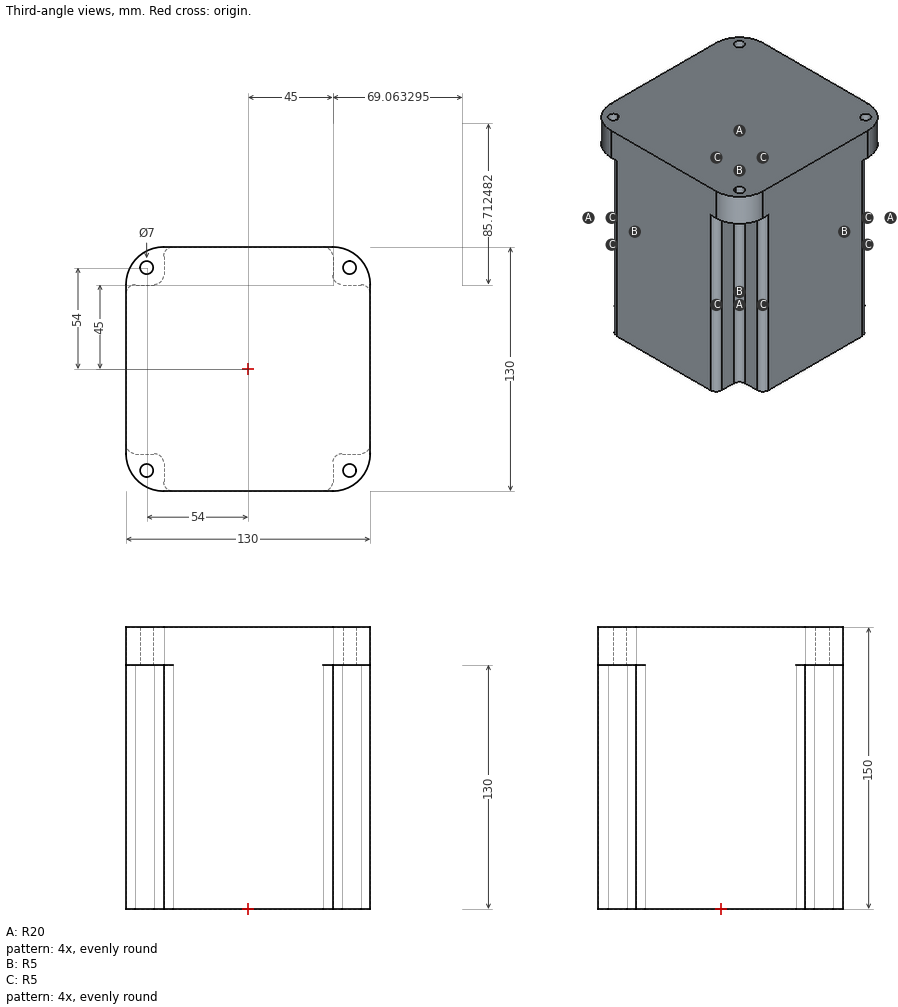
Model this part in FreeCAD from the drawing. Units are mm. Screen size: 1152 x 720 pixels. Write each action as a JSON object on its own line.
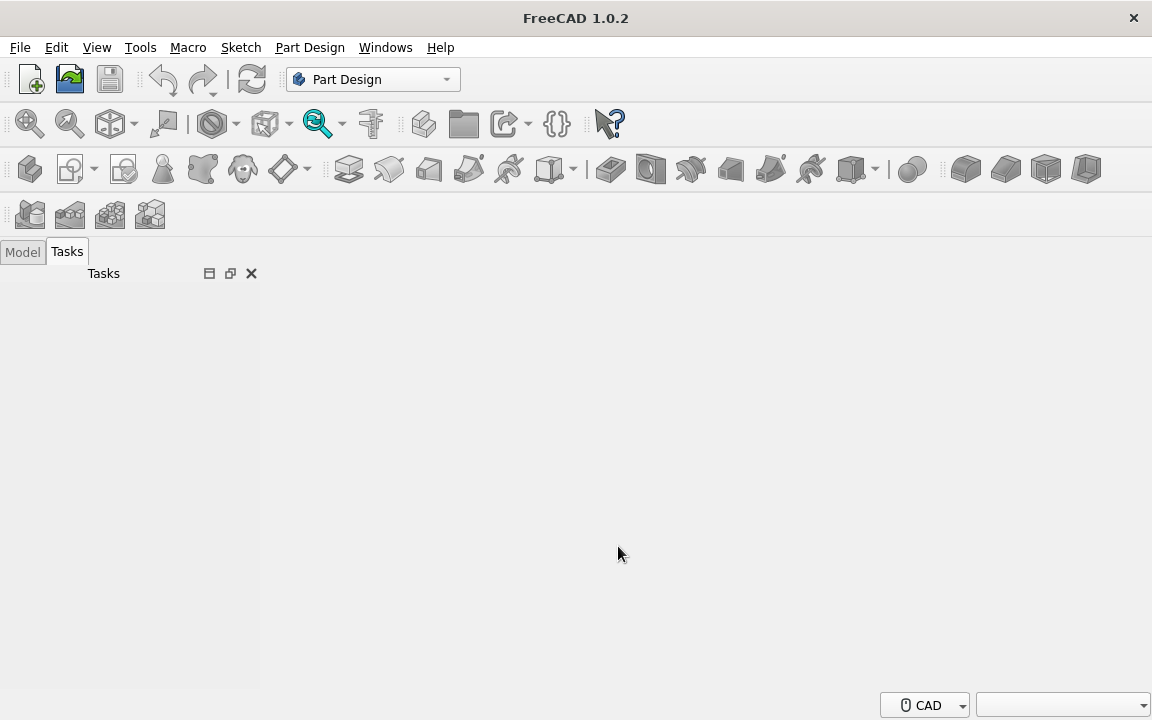
{"action": "key", "text": "ctrl+n"}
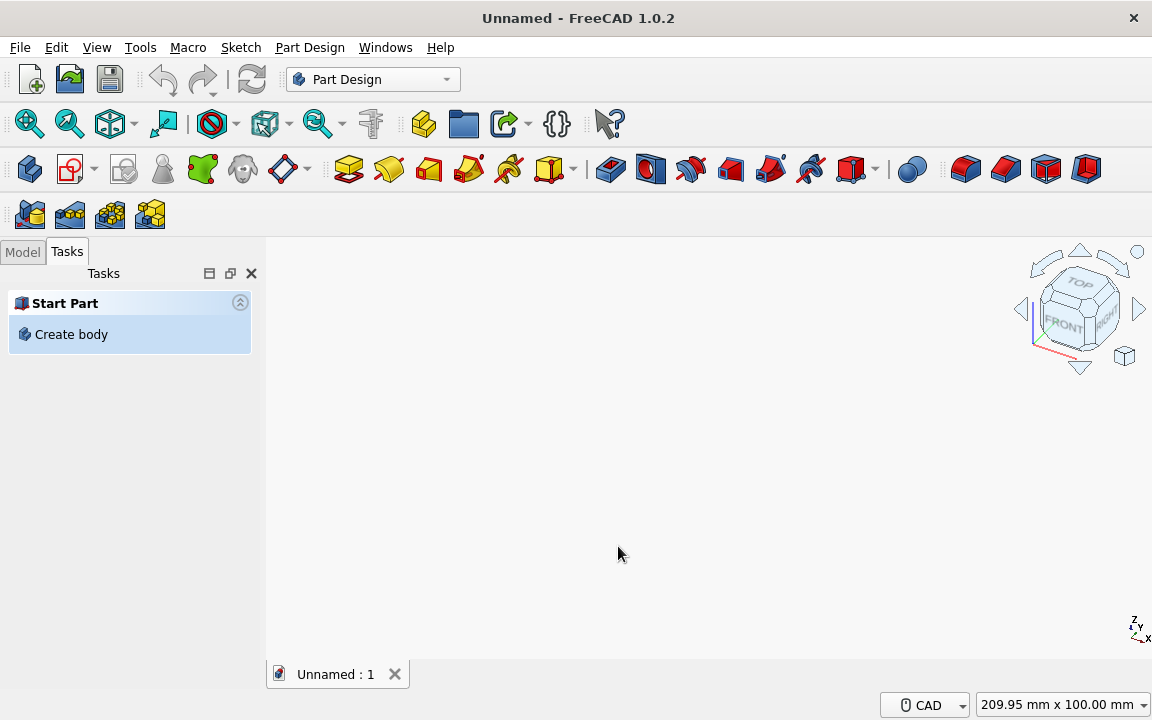
{"action": "left_click", "coordinate": [70, 170]}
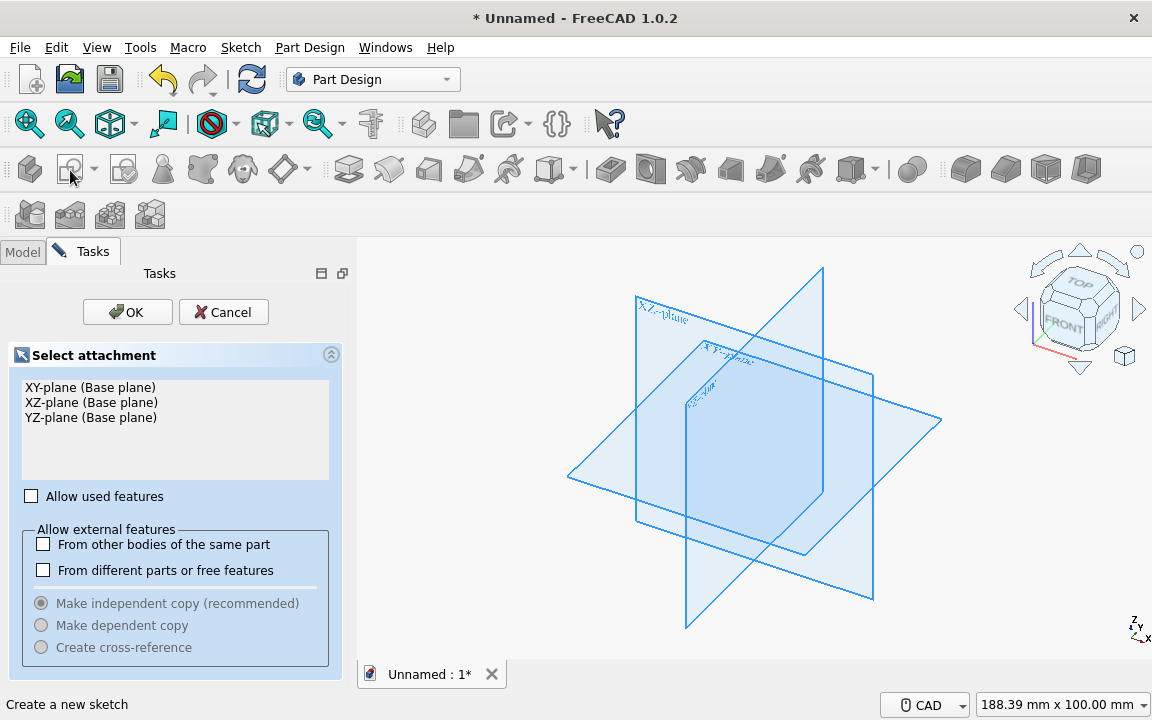
{"action": "left_click", "coordinate": [82, 388]}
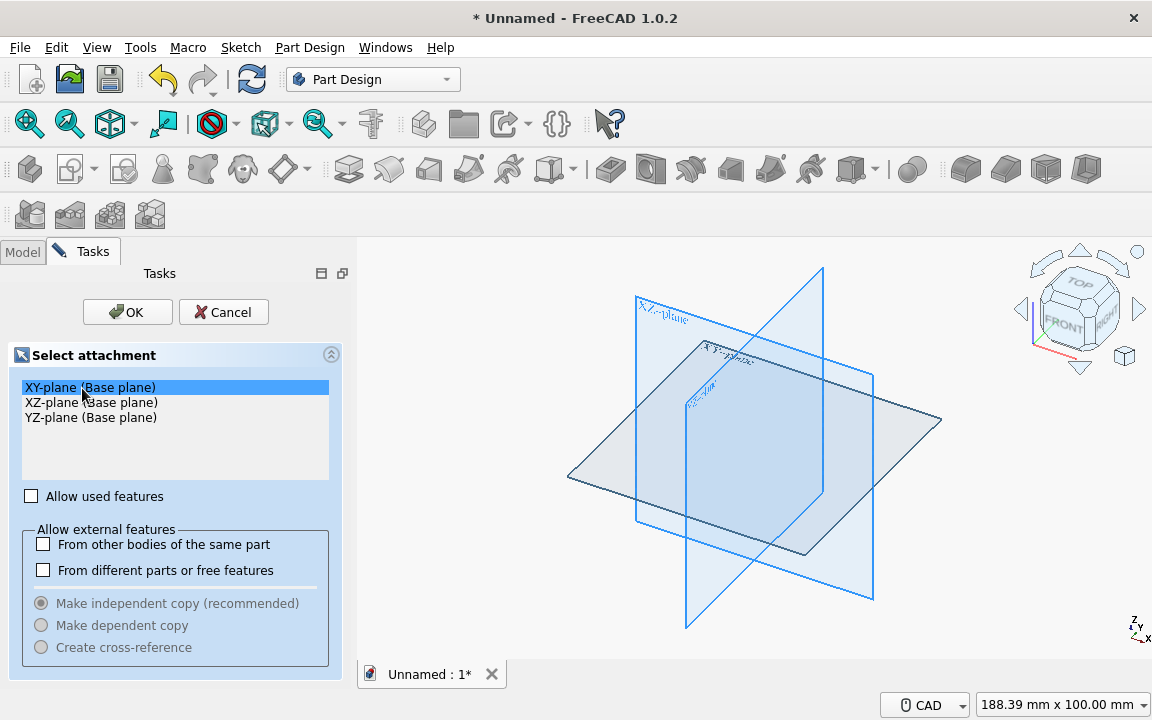
{"action": "left_click", "coordinate": [128, 312]}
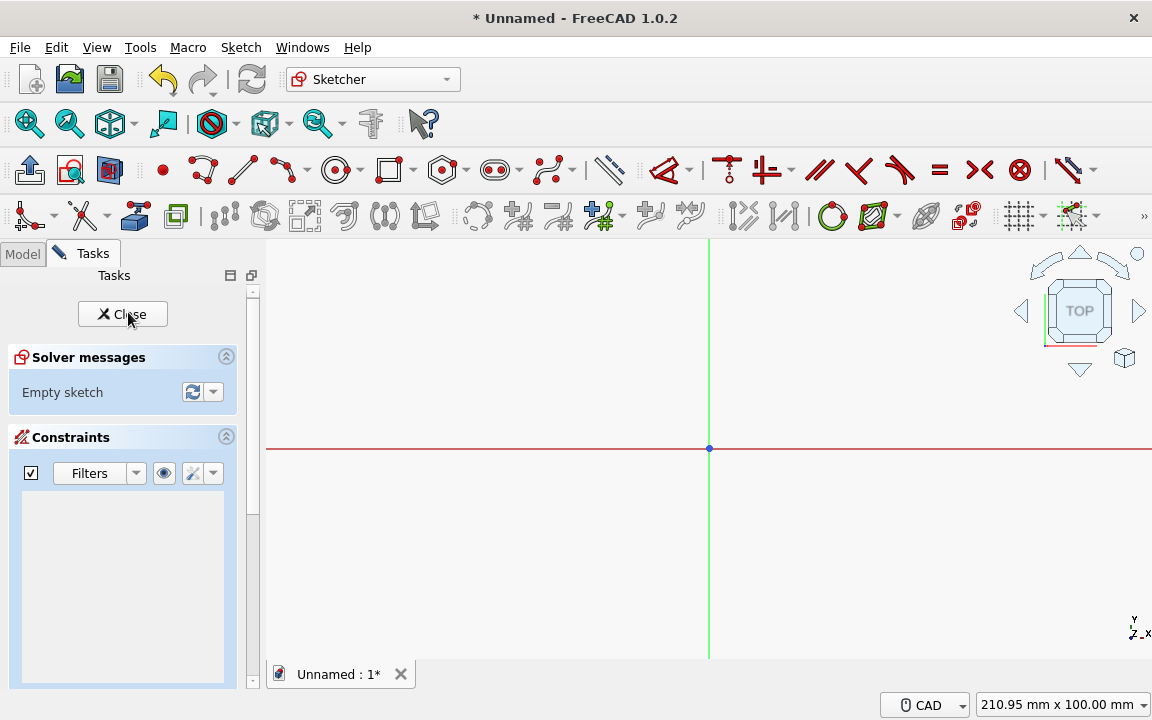
{"action": "scroll", "coordinate": [585, 449], "scroll_direction": "down", "scroll_amount": 4}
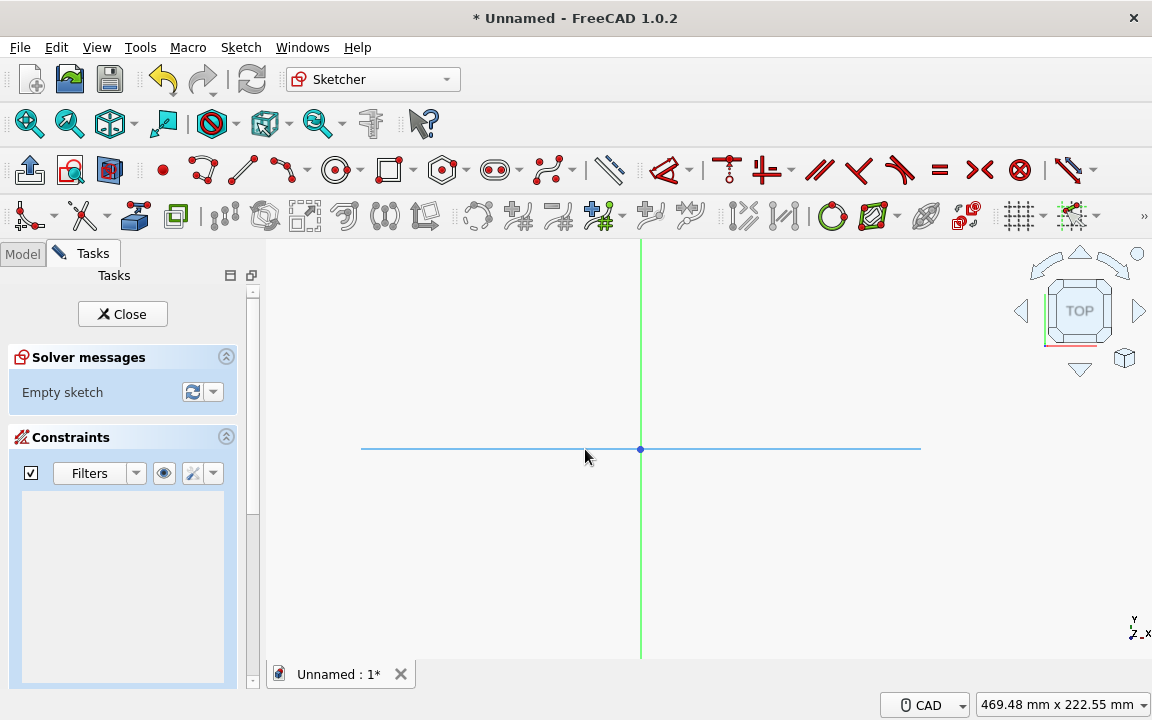
{"action": "key", "text": "g v"}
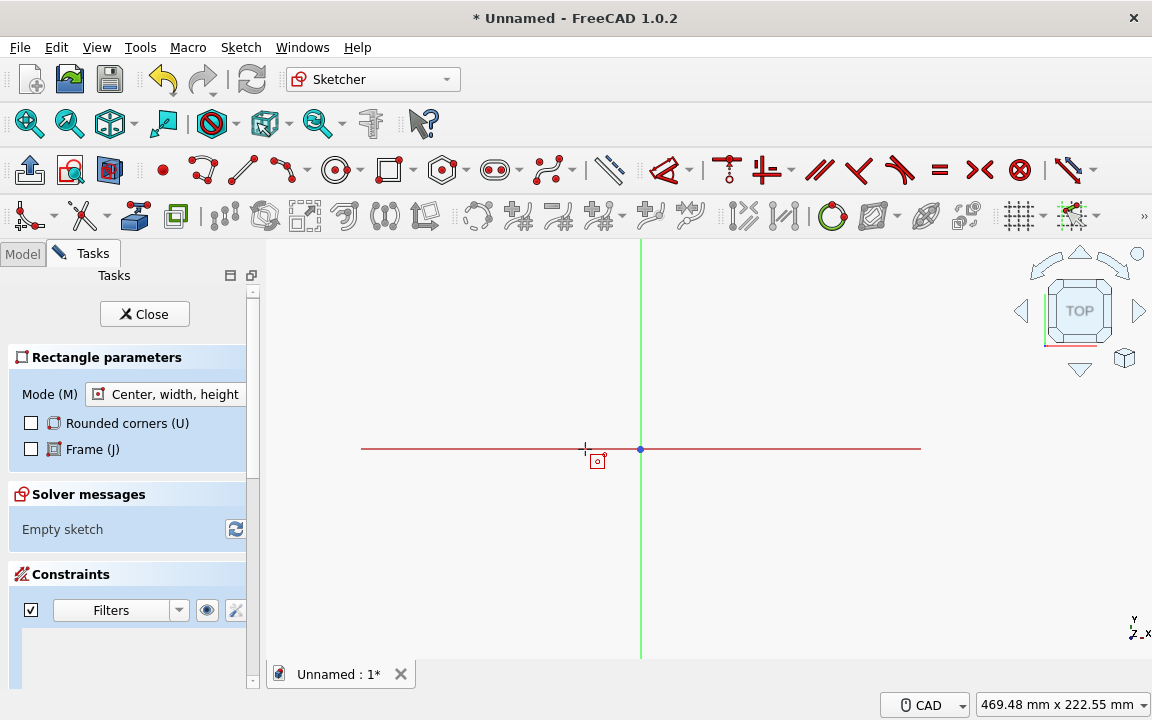
{"action": "left_click", "coordinate": [641, 449]}
{"action": "mouse_move", "coordinate": [764, 327]}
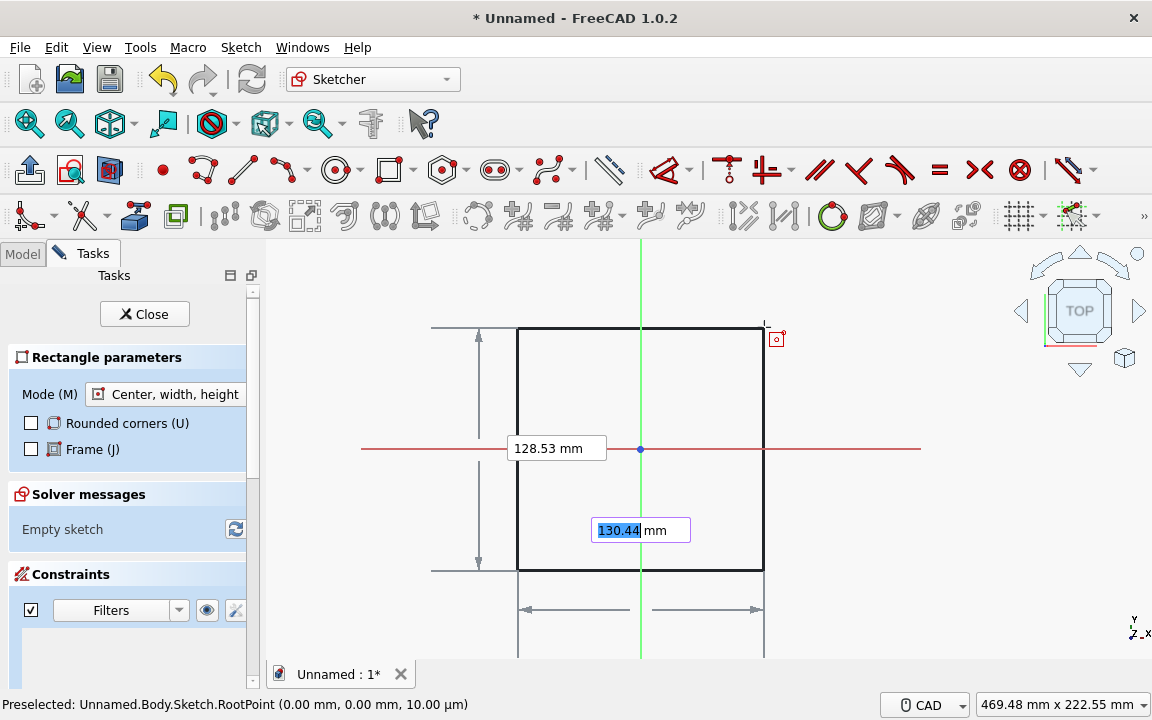
{"action": "type", "text": "130"}
{"action": "key", "text": "Tab"}
{"action": "type", "text": "130"}
{"action": "key", "text": "Return"}
{"action": "key", "text": "Escape"}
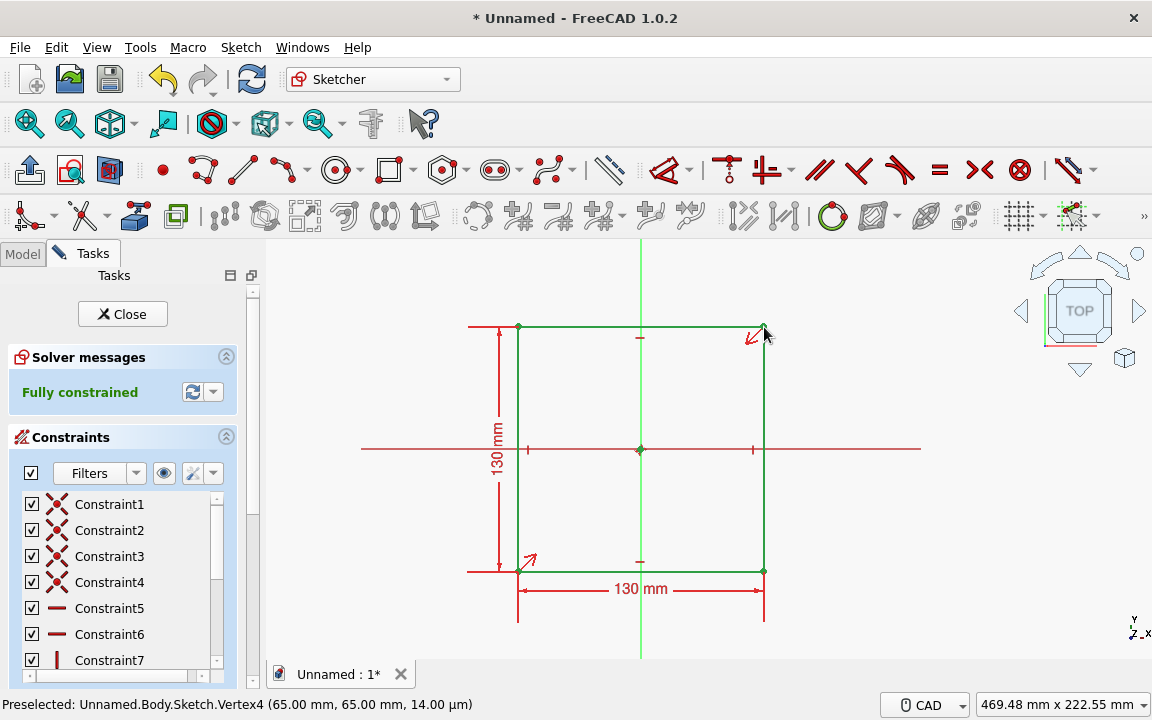
{"action": "left_click", "coordinate": [123, 314]}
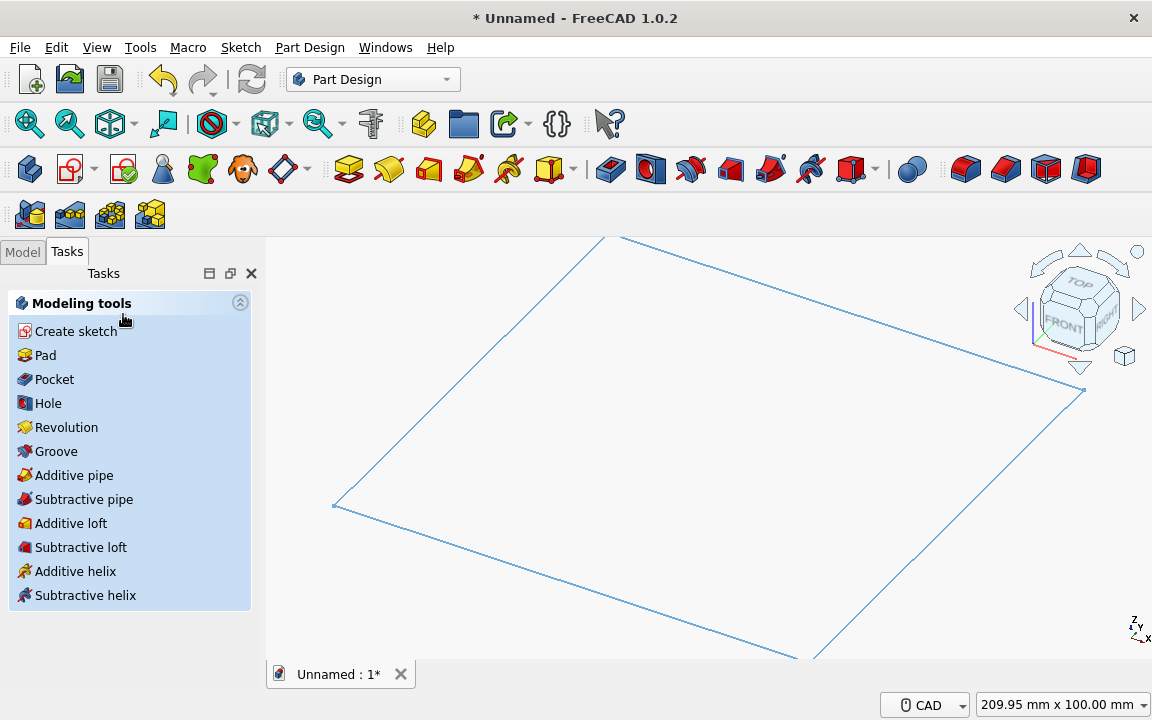
{"action": "left_click", "coordinate": [350, 170]}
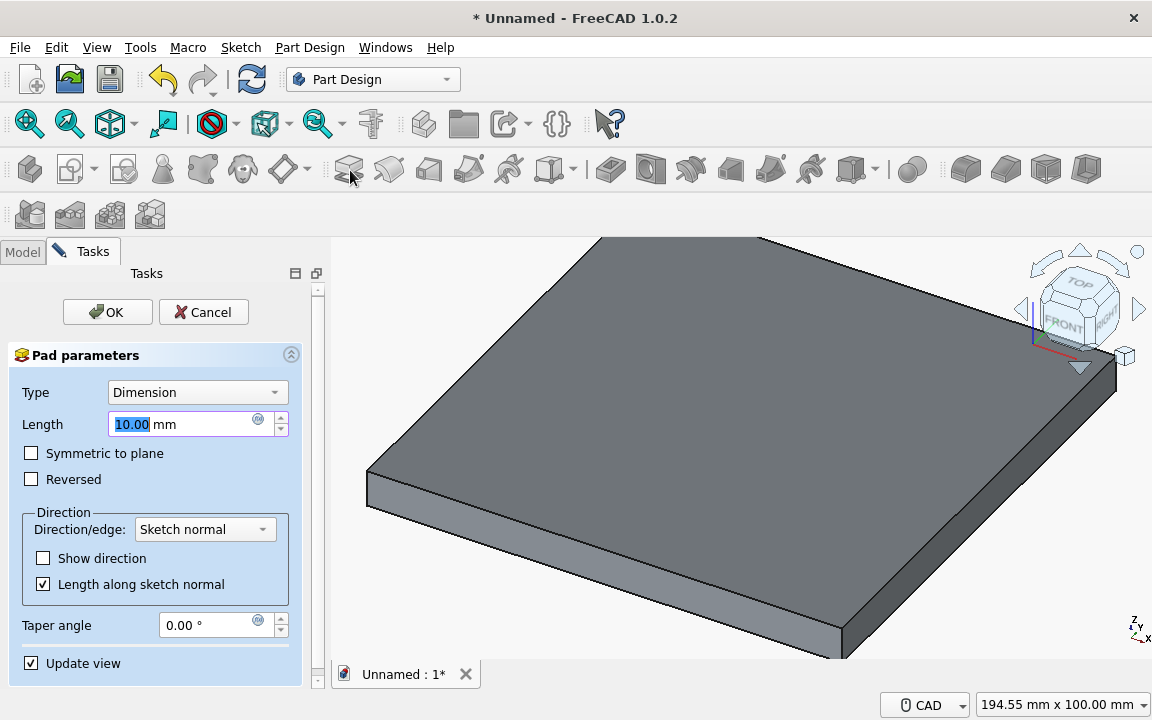
{"action": "type", "text": "150"}
{"action": "key", "text": "Tab"}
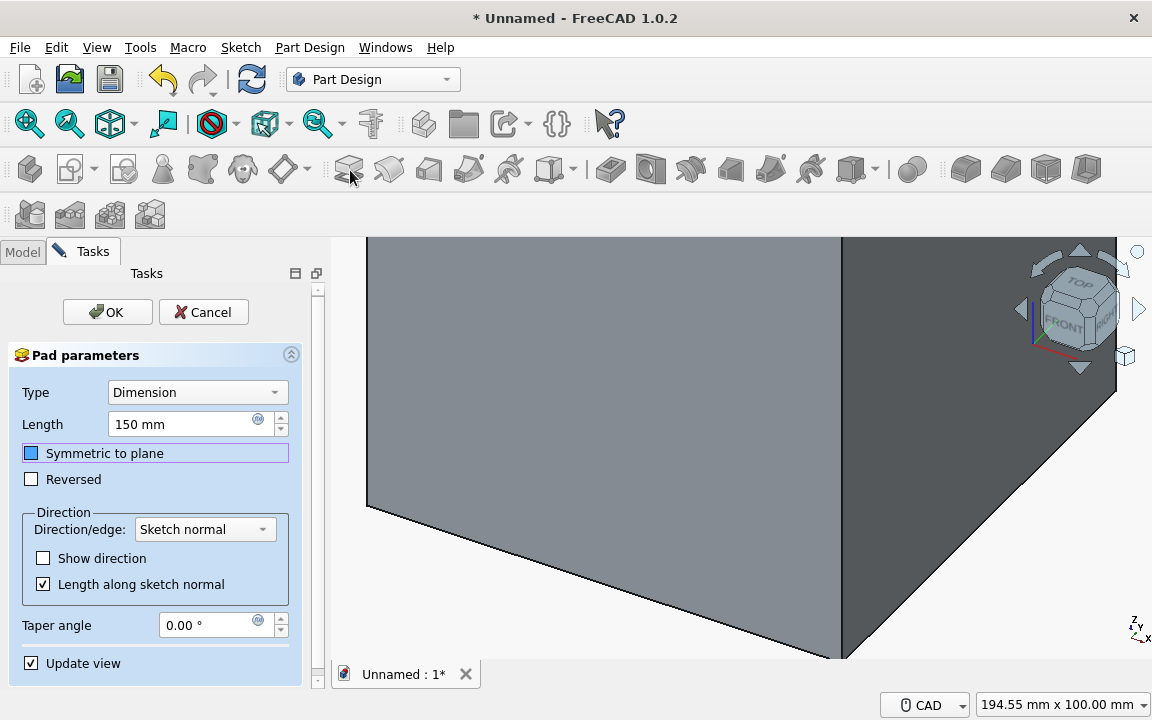
{"action": "left_click", "coordinate": [108, 312]}